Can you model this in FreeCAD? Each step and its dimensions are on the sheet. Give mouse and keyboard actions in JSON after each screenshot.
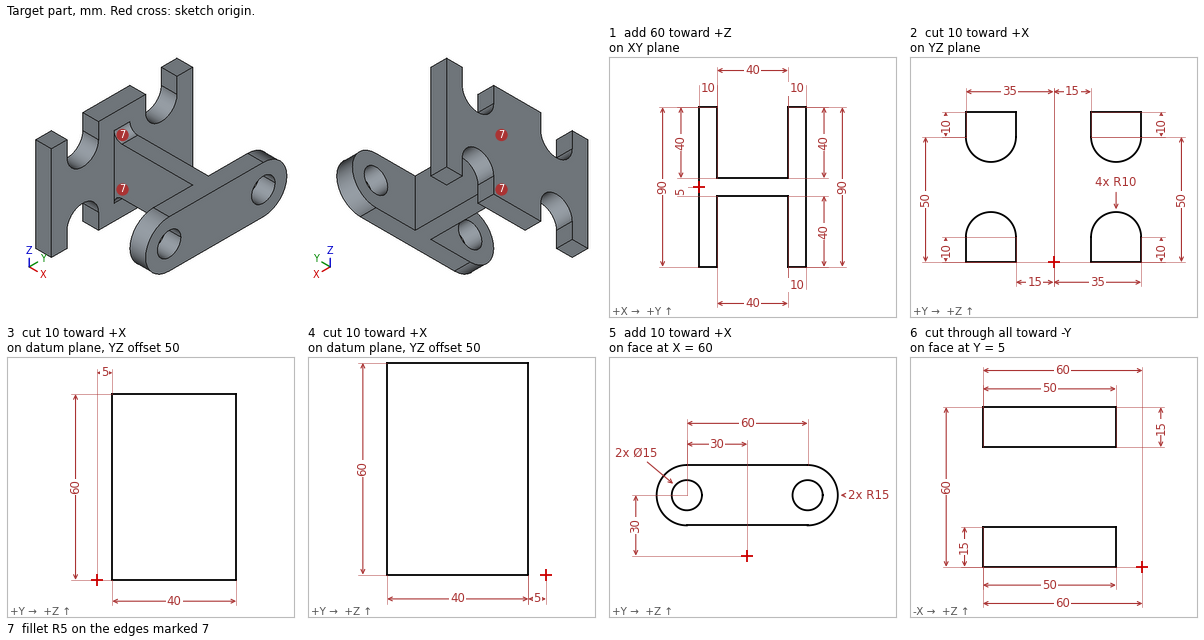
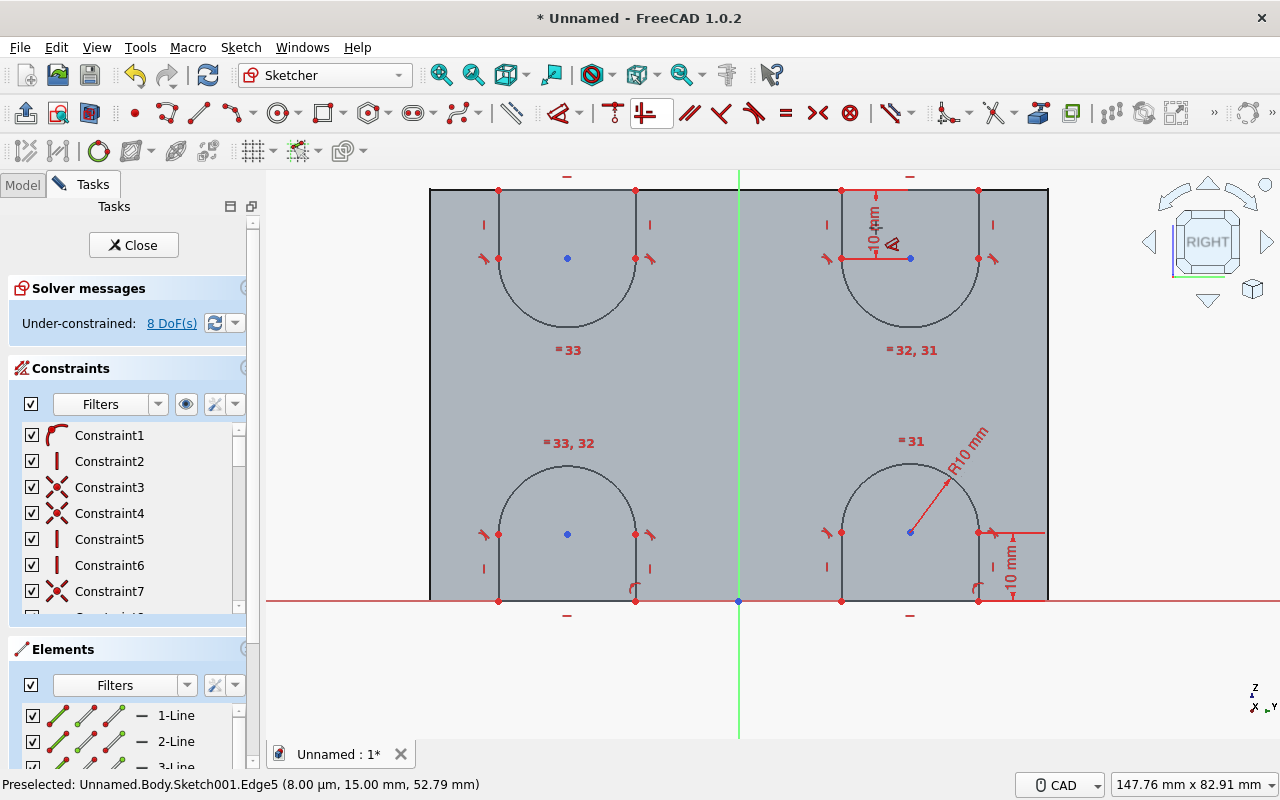
{"action": "left_click", "coordinate": [636, 555]}
{"action": "left_click", "coordinate": [602, 568]}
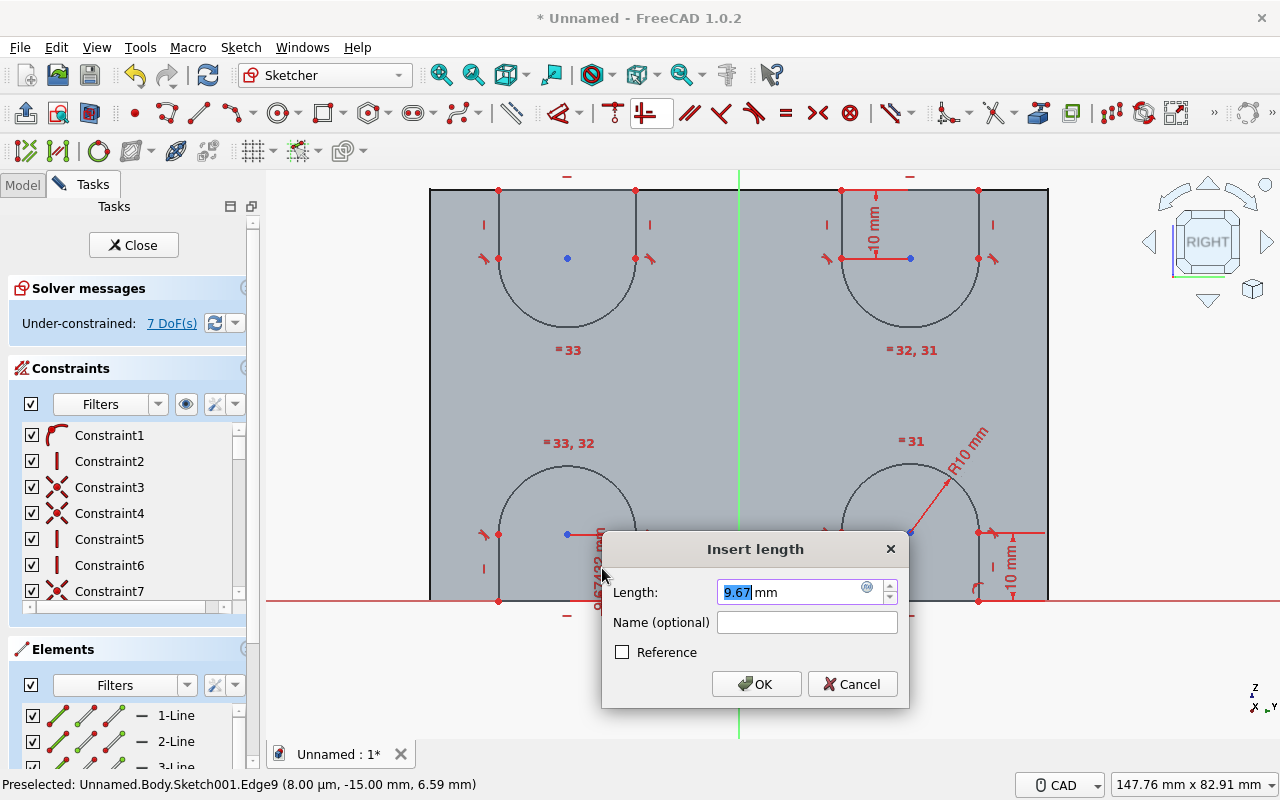
{"action": "type", "text": "10"}
{"action": "key", "text": "Return"}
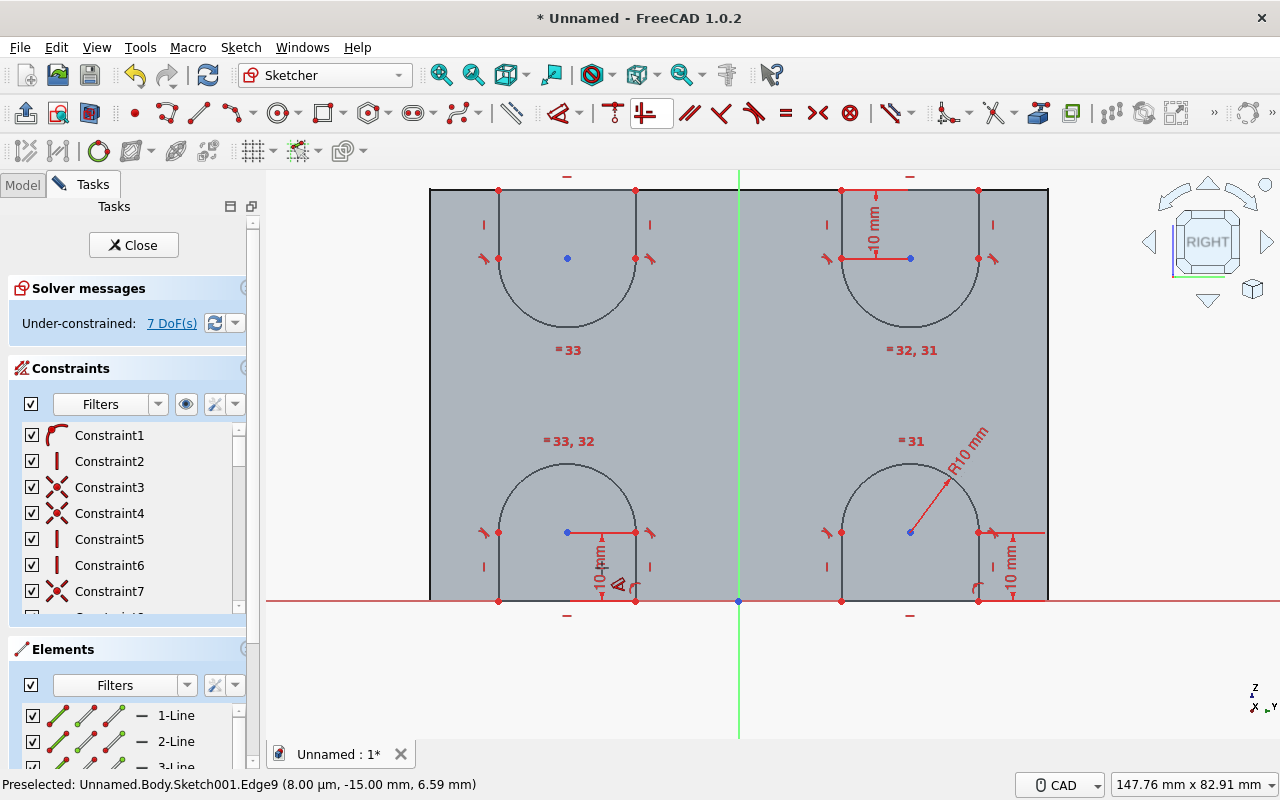
{"action": "left_click", "coordinate": [499, 238]}
{"action": "left_click", "coordinate": [465, 228]}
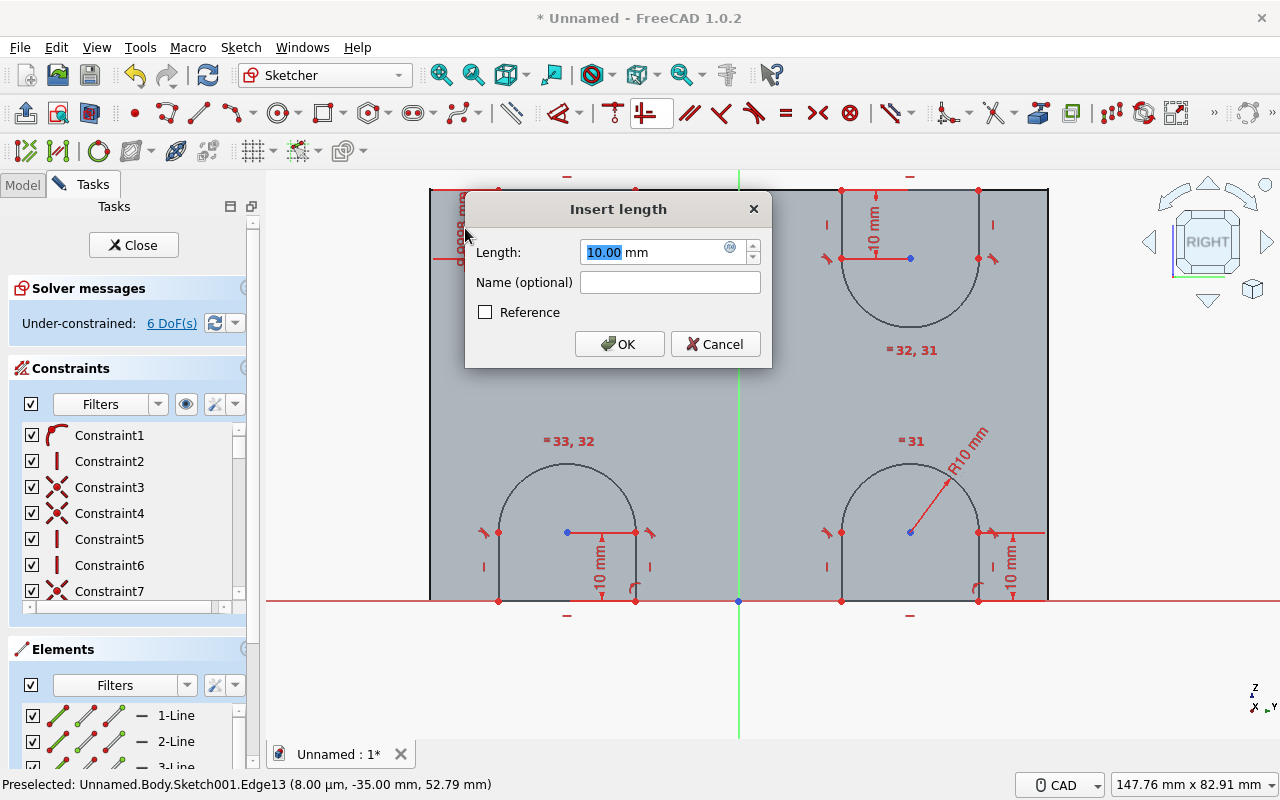
{"action": "type", "text": "10"}
{"action": "key", "text": "Return"}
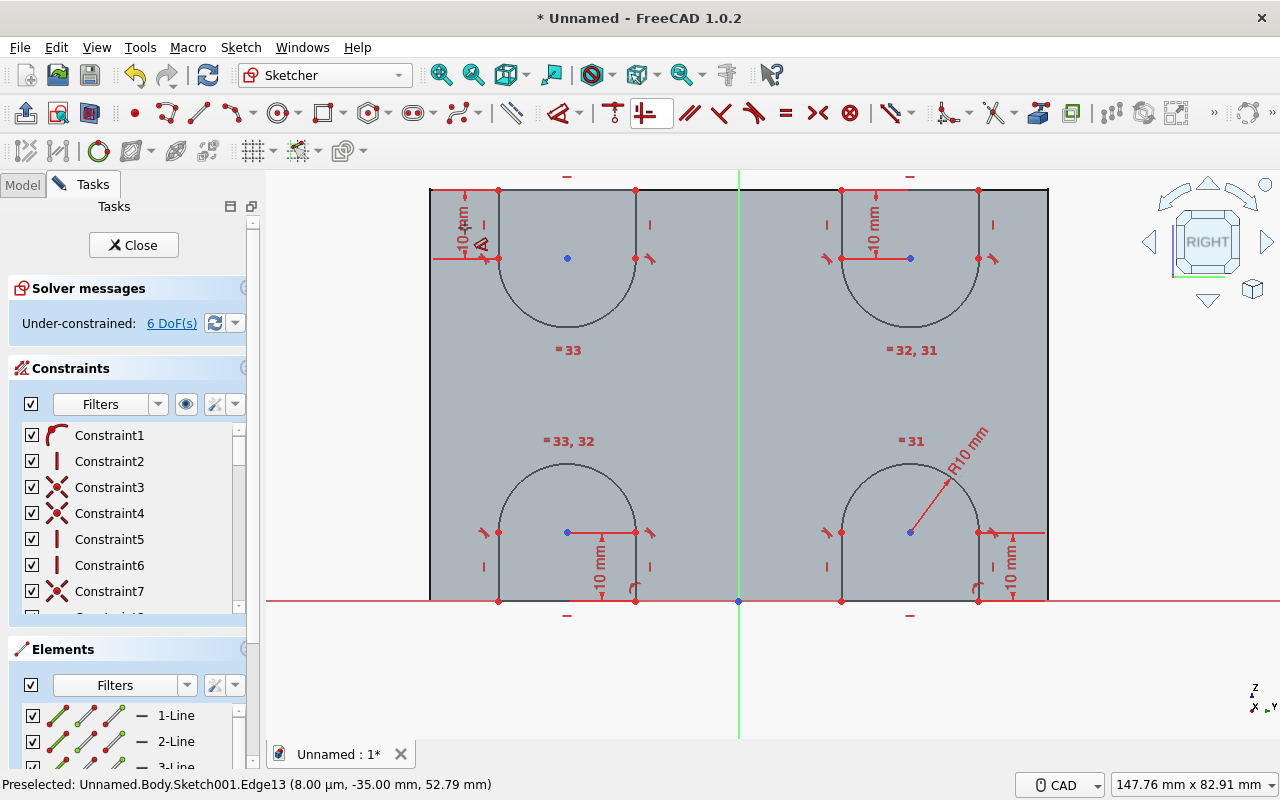
{"action": "left_click", "coordinate": [979, 533]}
{"action": "left_click", "coordinate": [859, 635]}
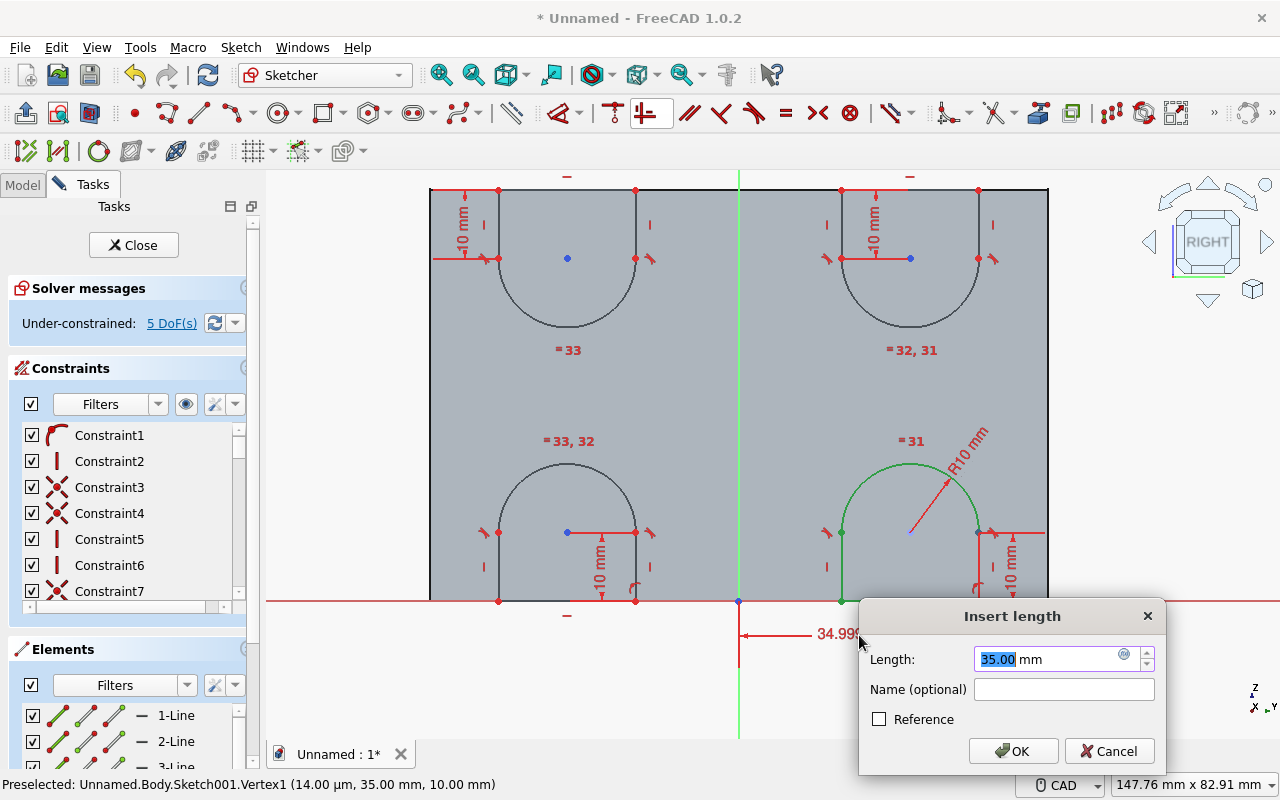
{"action": "type", "text": "35"}
{"action": "key", "text": "Return"}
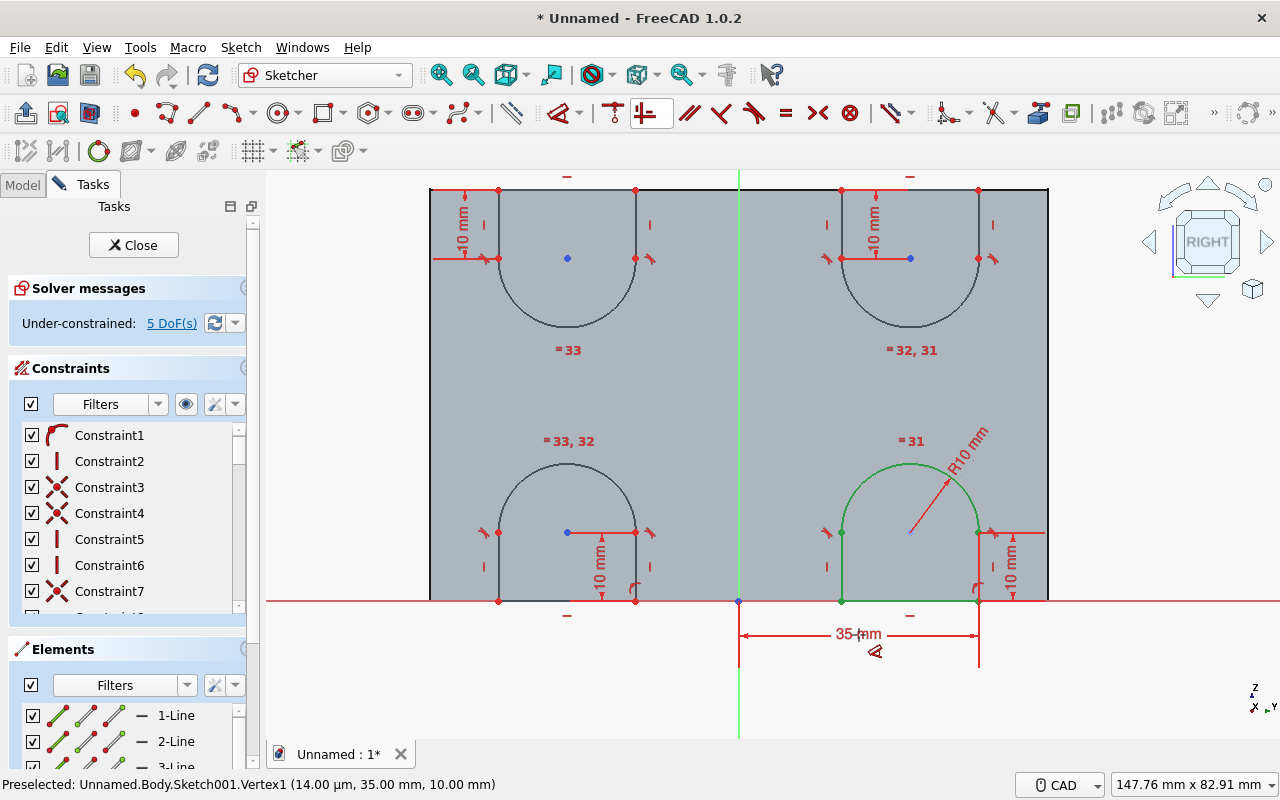
{"action": "left_click", "coordinate": [842, 259]}
{"action": "left_click", "coordinate": [767, 635]}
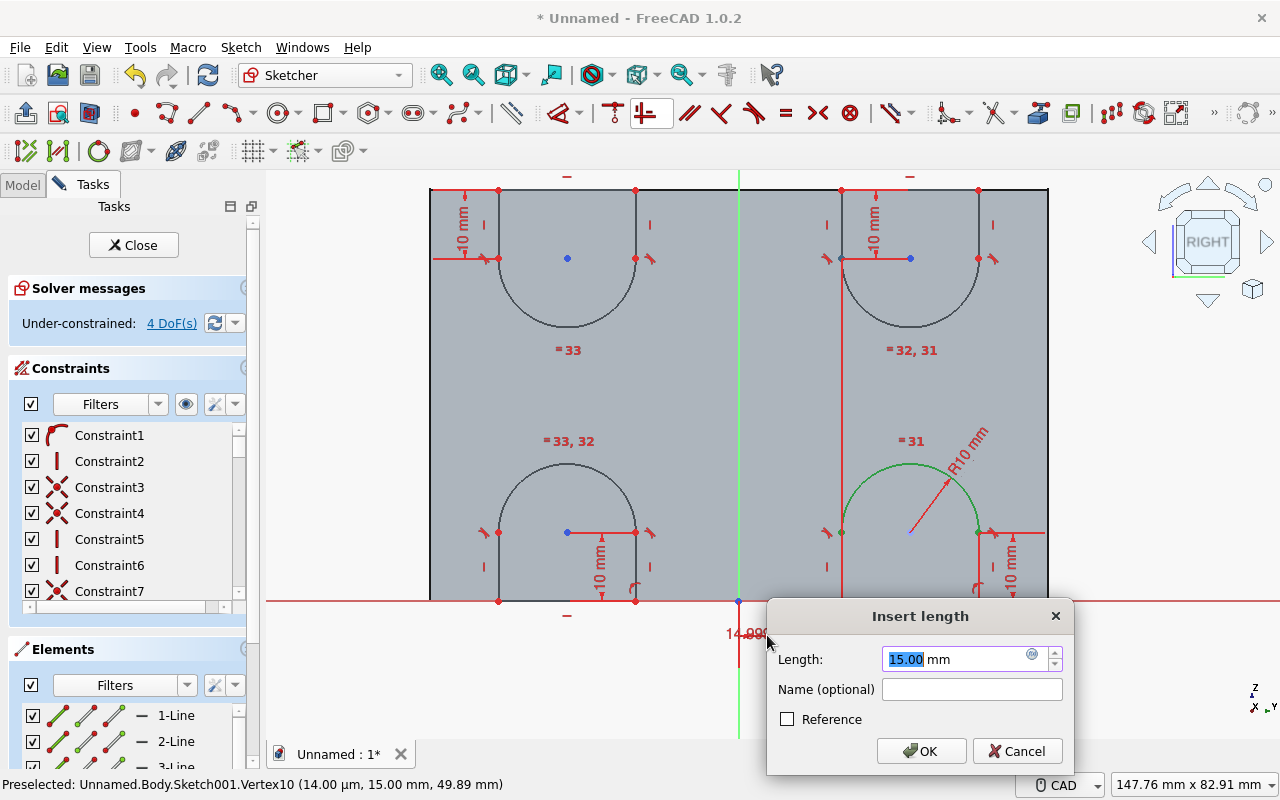
{"action": "type", "text": "15"}
{"action": "key", "text": "Return"}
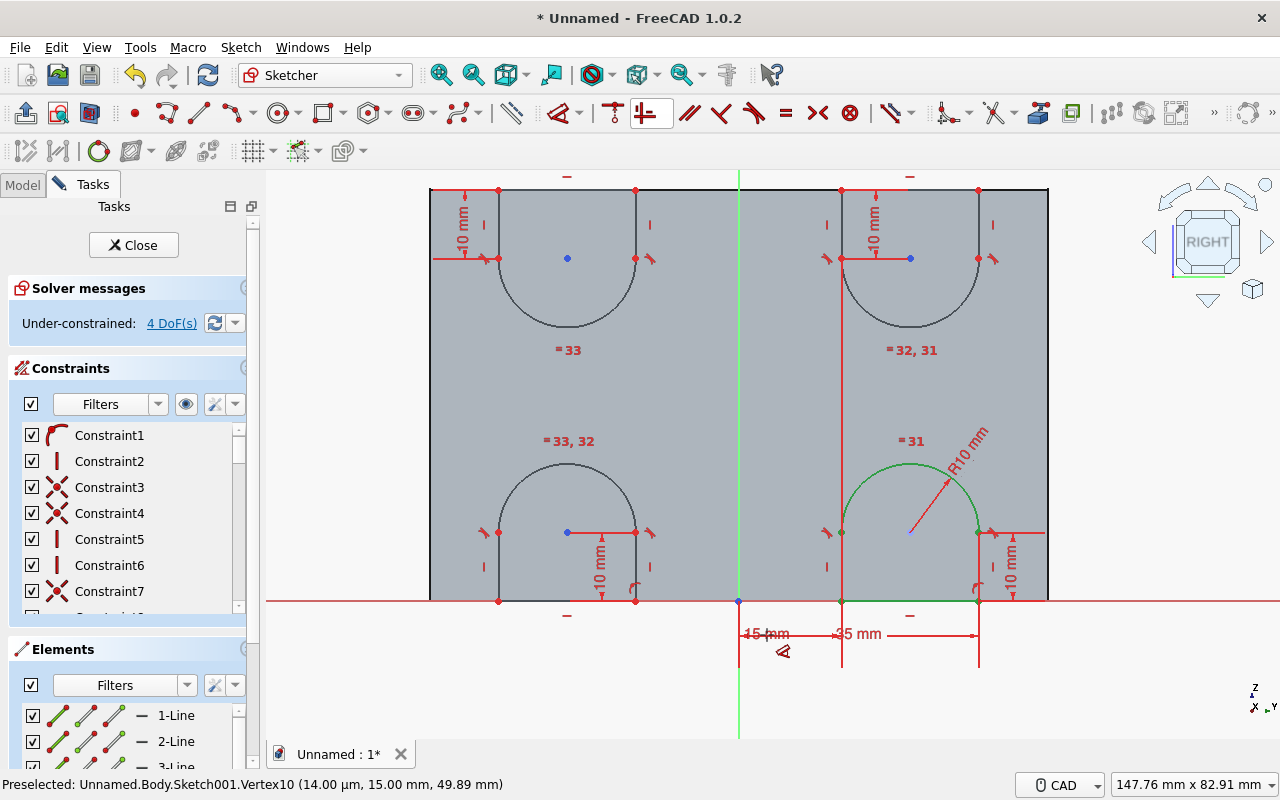
{"action": "left_click", "coordinate": [842, 259]}
{"action": "left_click", "coordinate": [876, 430]}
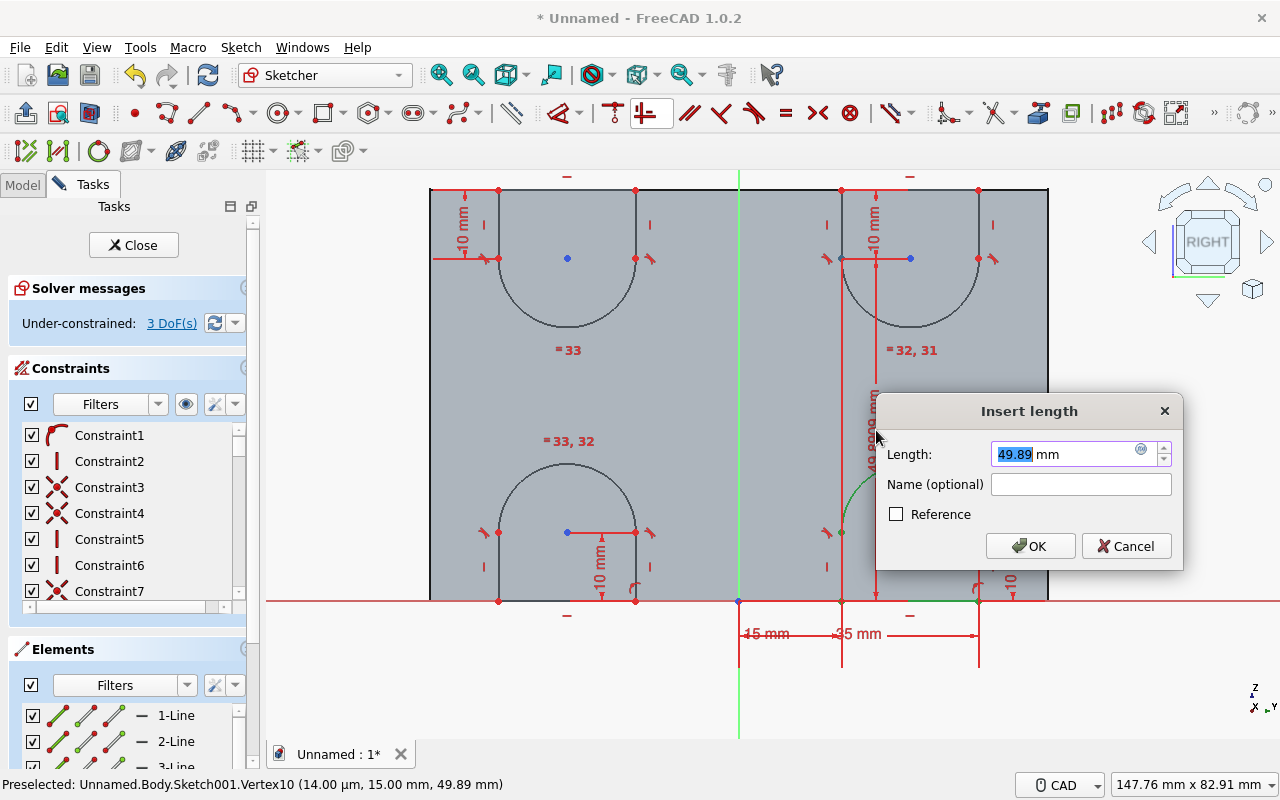
{"action": "type", "text": "50"}
{"action": "key", "text": "Return"}